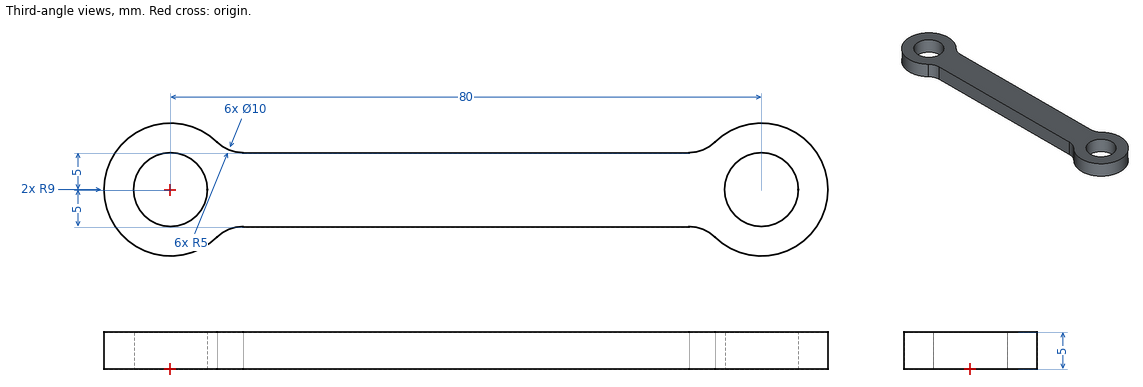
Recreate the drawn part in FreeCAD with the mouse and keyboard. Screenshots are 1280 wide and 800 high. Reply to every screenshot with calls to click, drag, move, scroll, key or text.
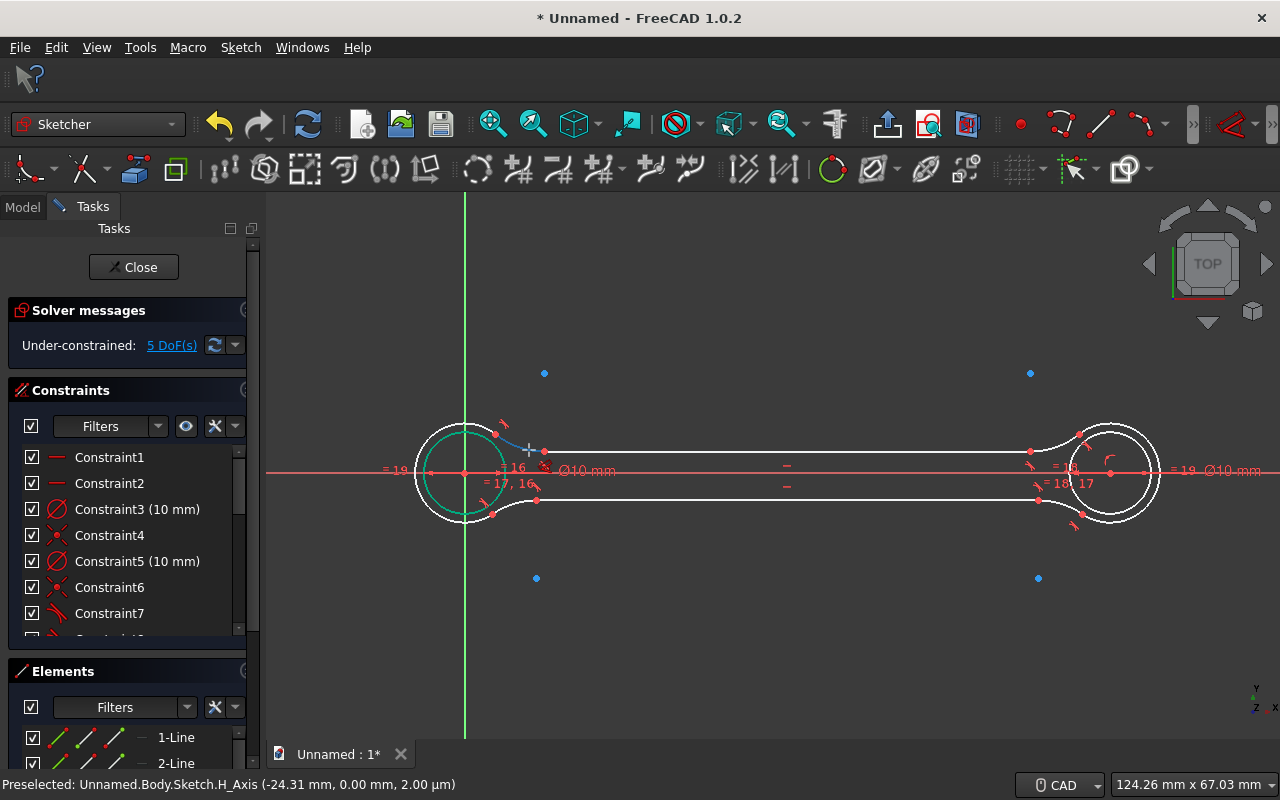
click(529, 450)
click(442, 413)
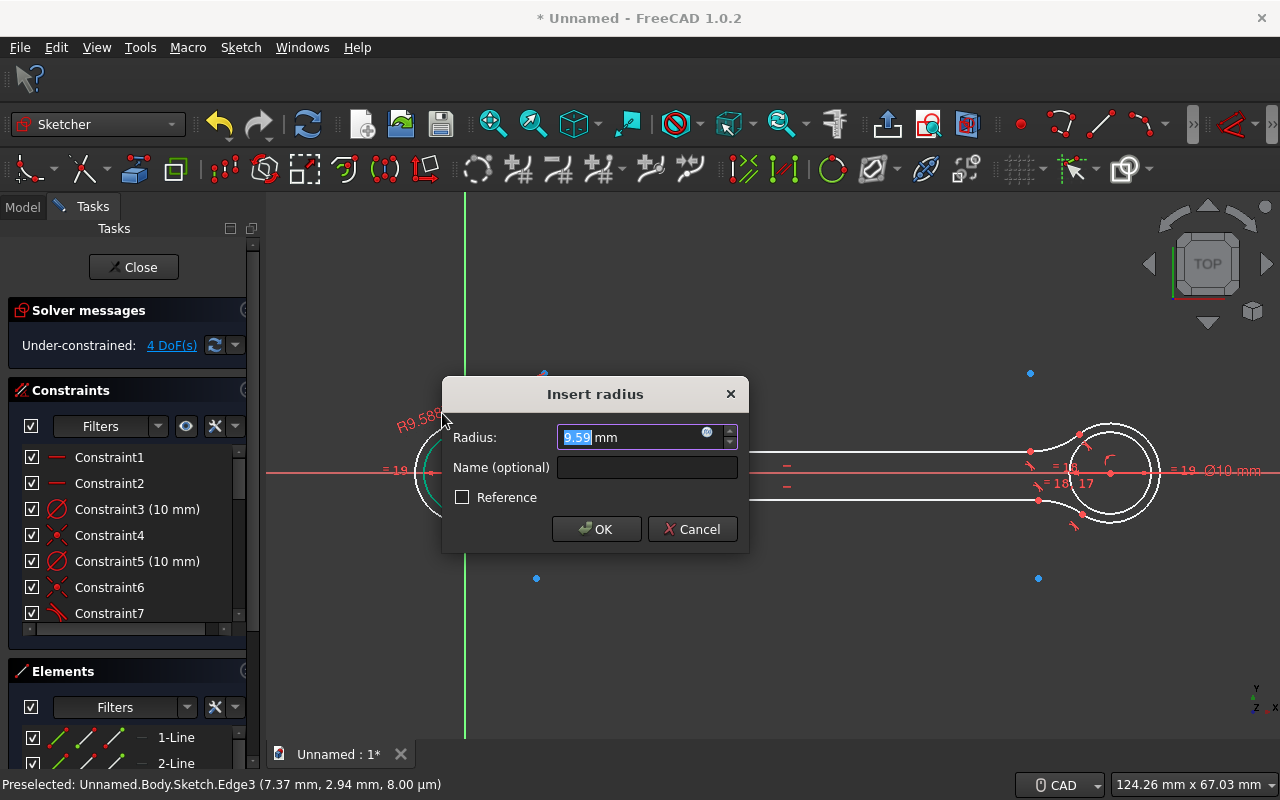
text(5)
key(Return)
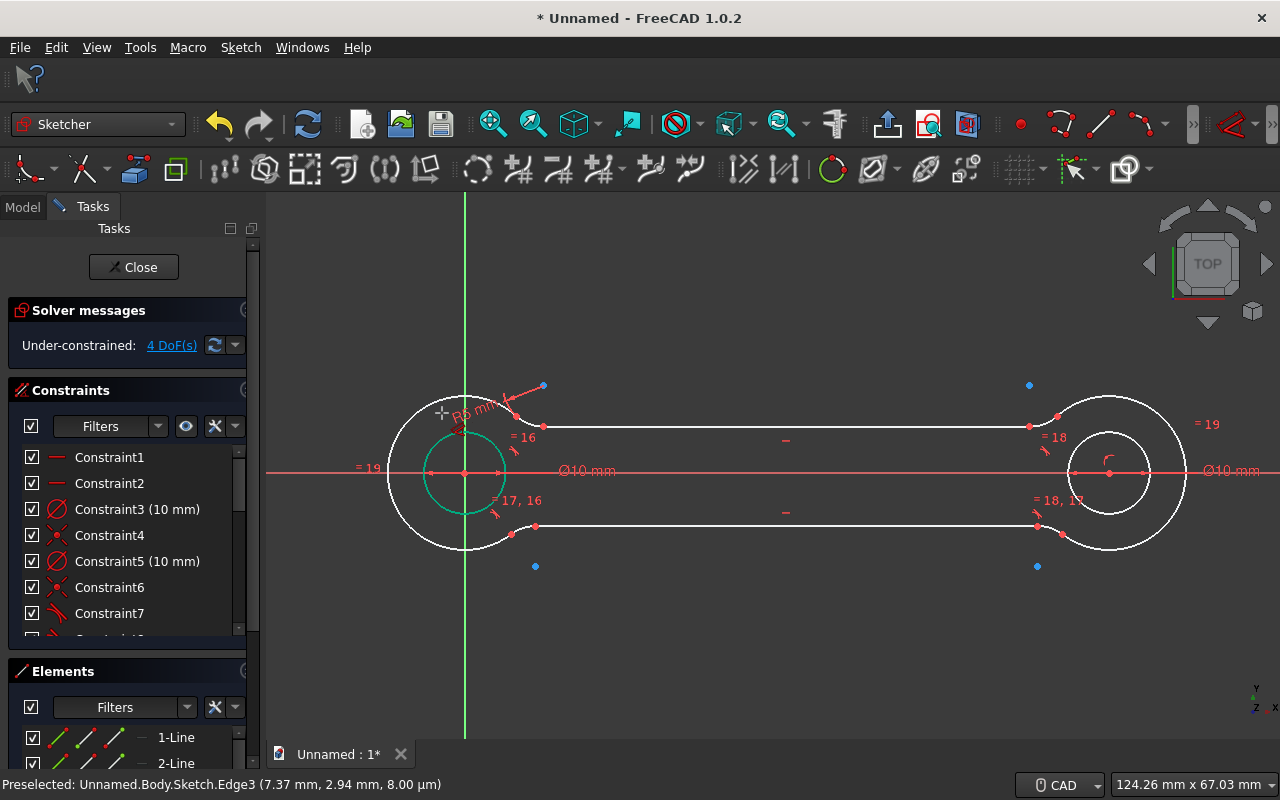
click(420, 411)
click(401, 385)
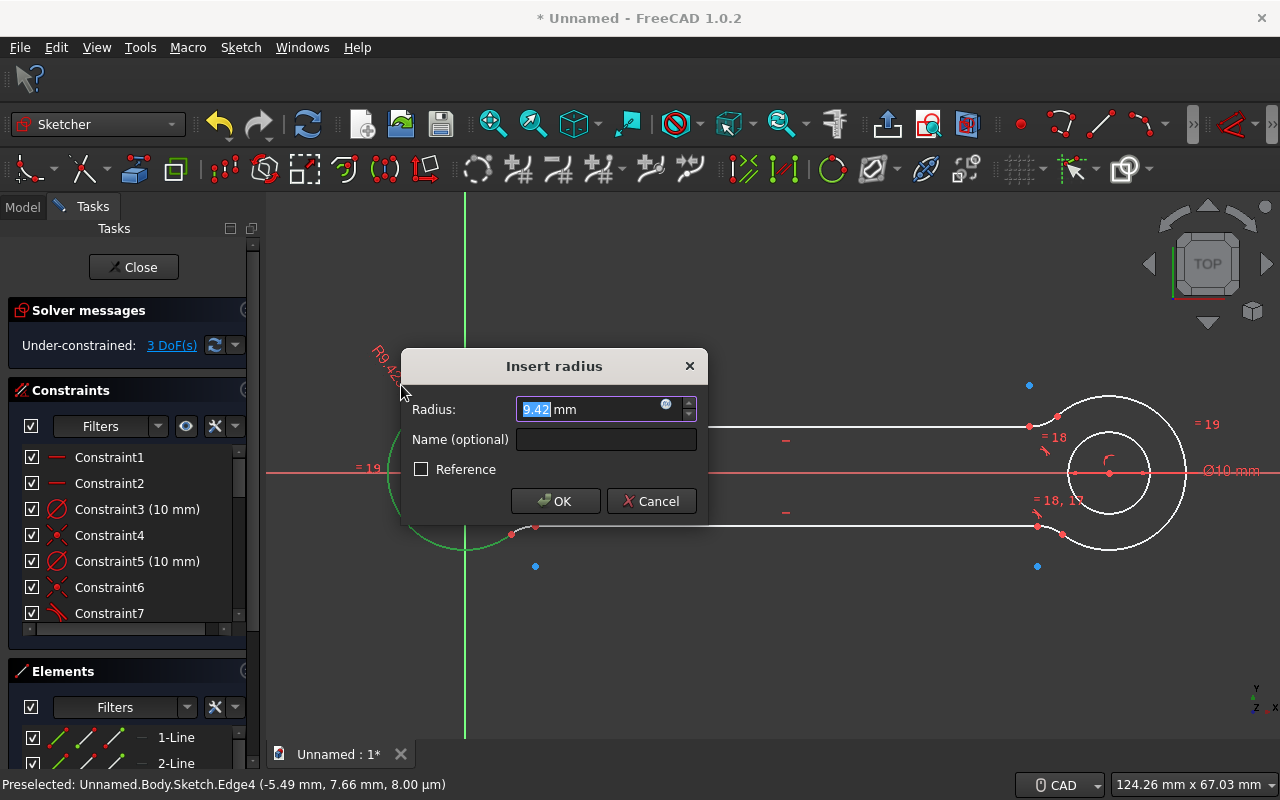
text(9)
key(Return)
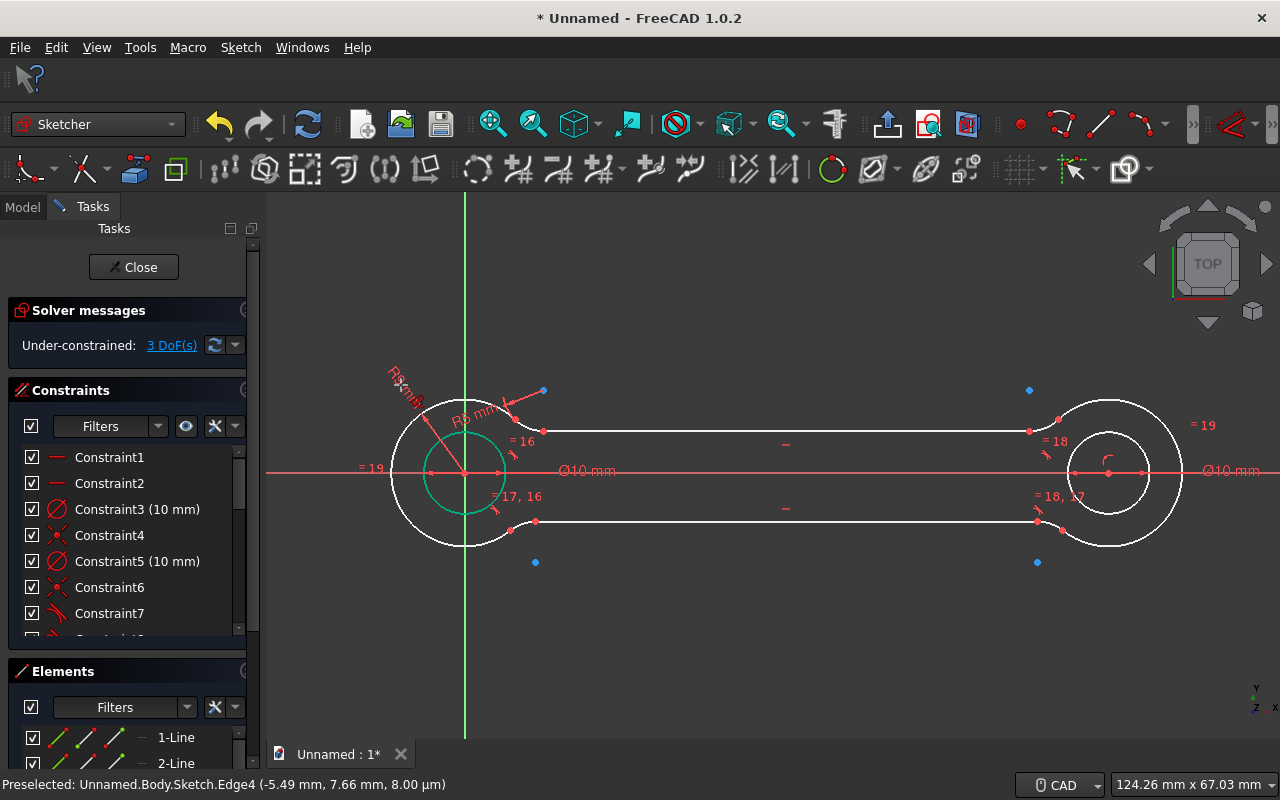
click(1030, 431)
click(1064, 442)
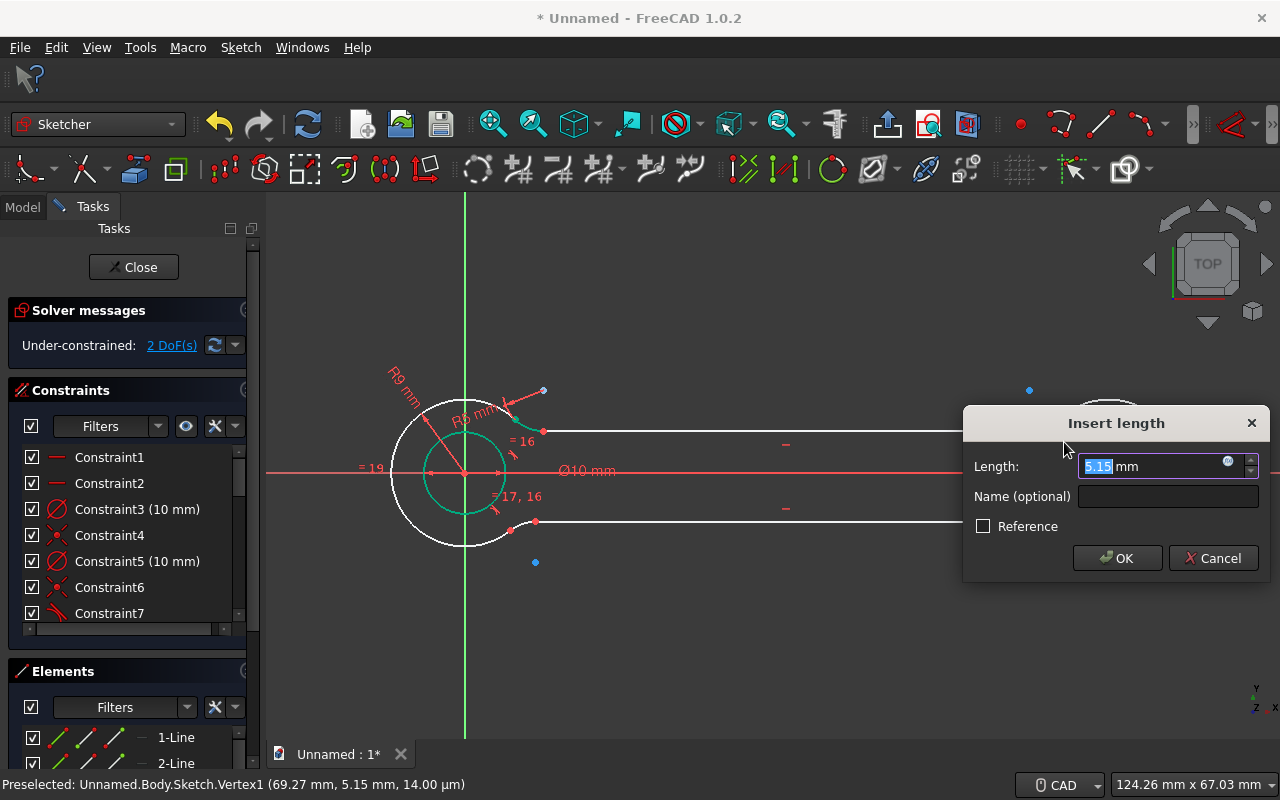
text(5)
key(Return)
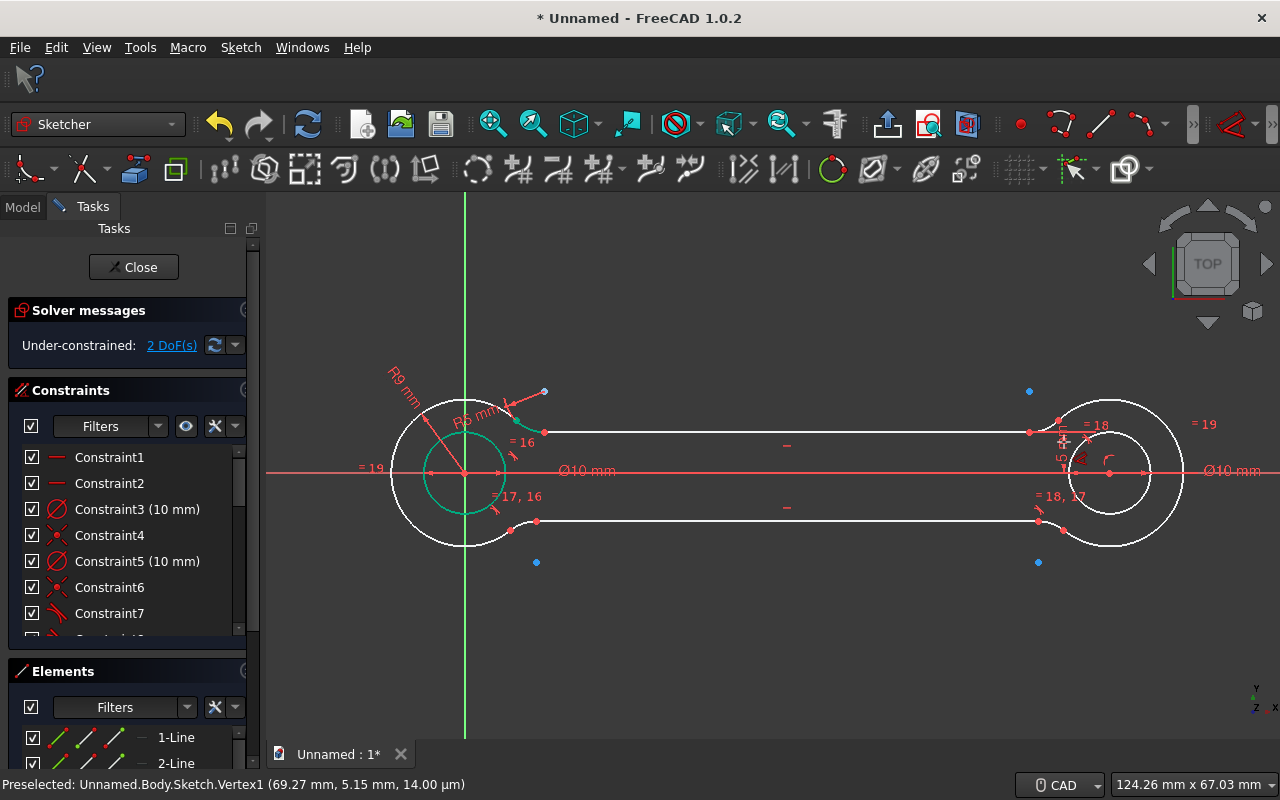
click(536, 521)
click(570, 497)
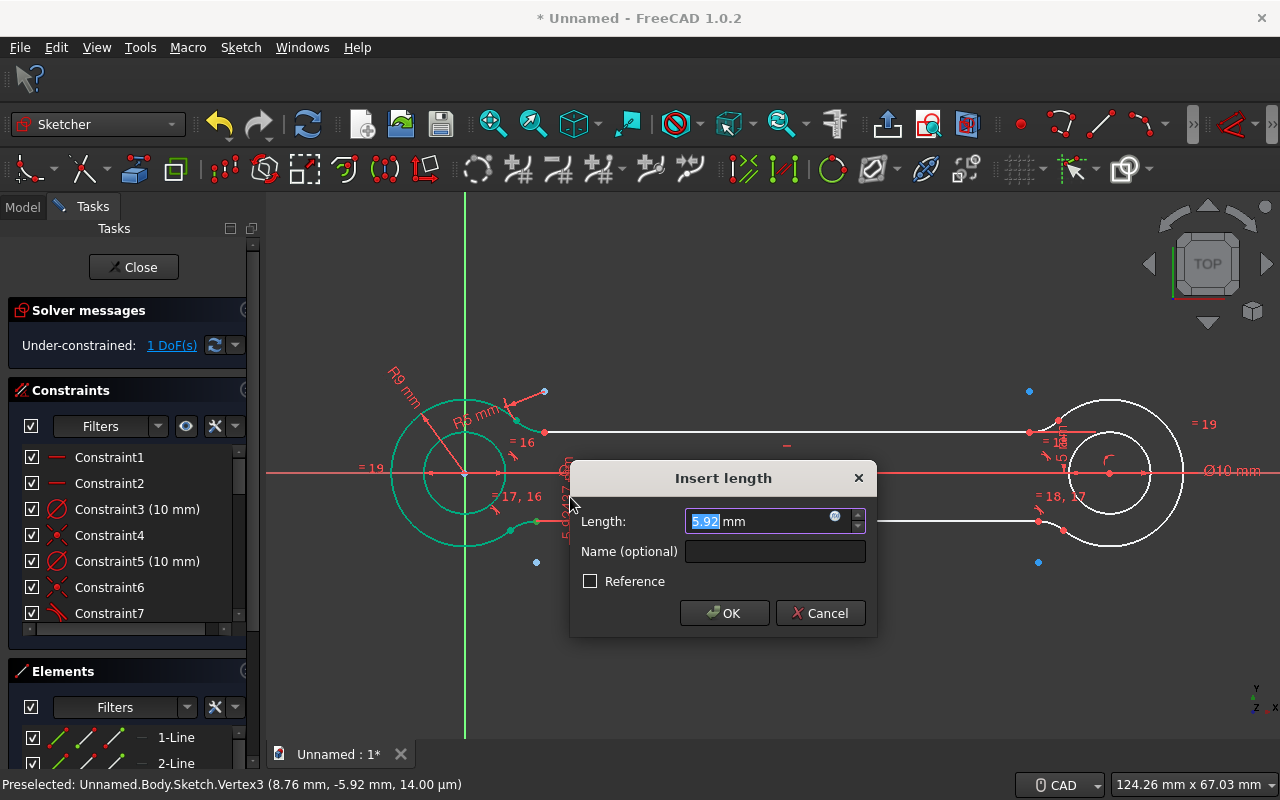
text(5)
key(Return)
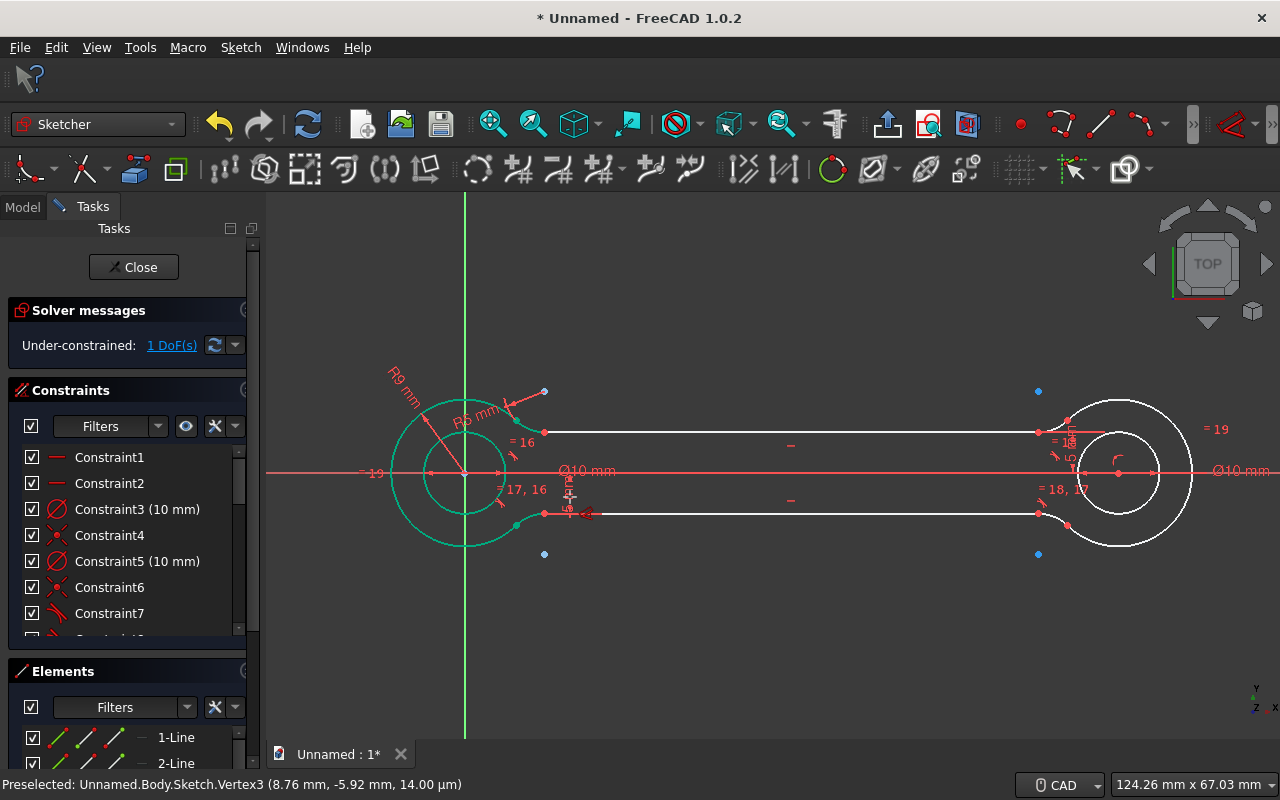
scroll(528, 450, down, 2)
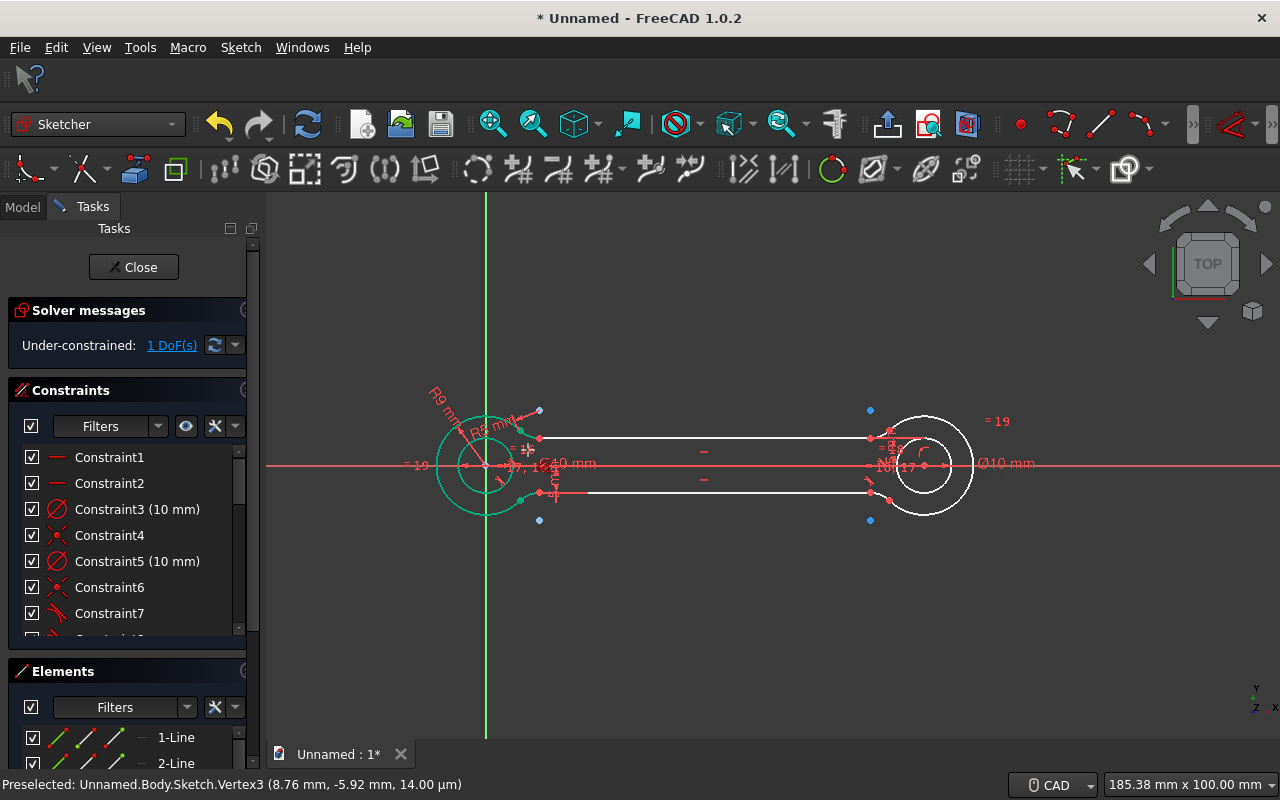
click(924, 466)
click(705, 524)